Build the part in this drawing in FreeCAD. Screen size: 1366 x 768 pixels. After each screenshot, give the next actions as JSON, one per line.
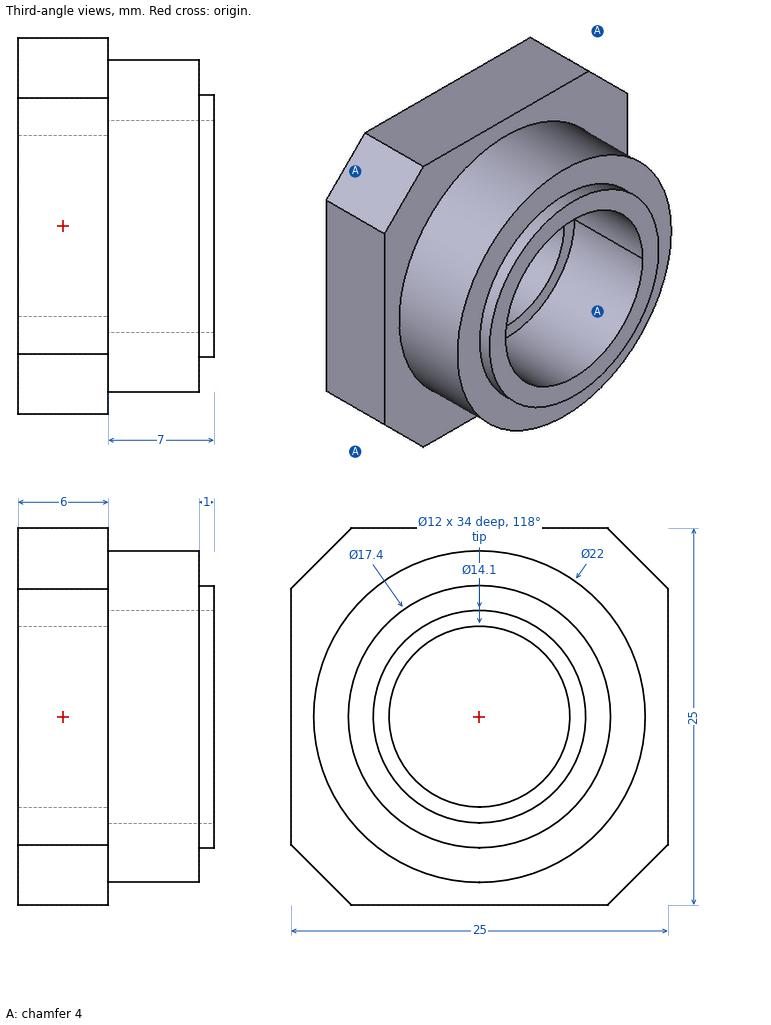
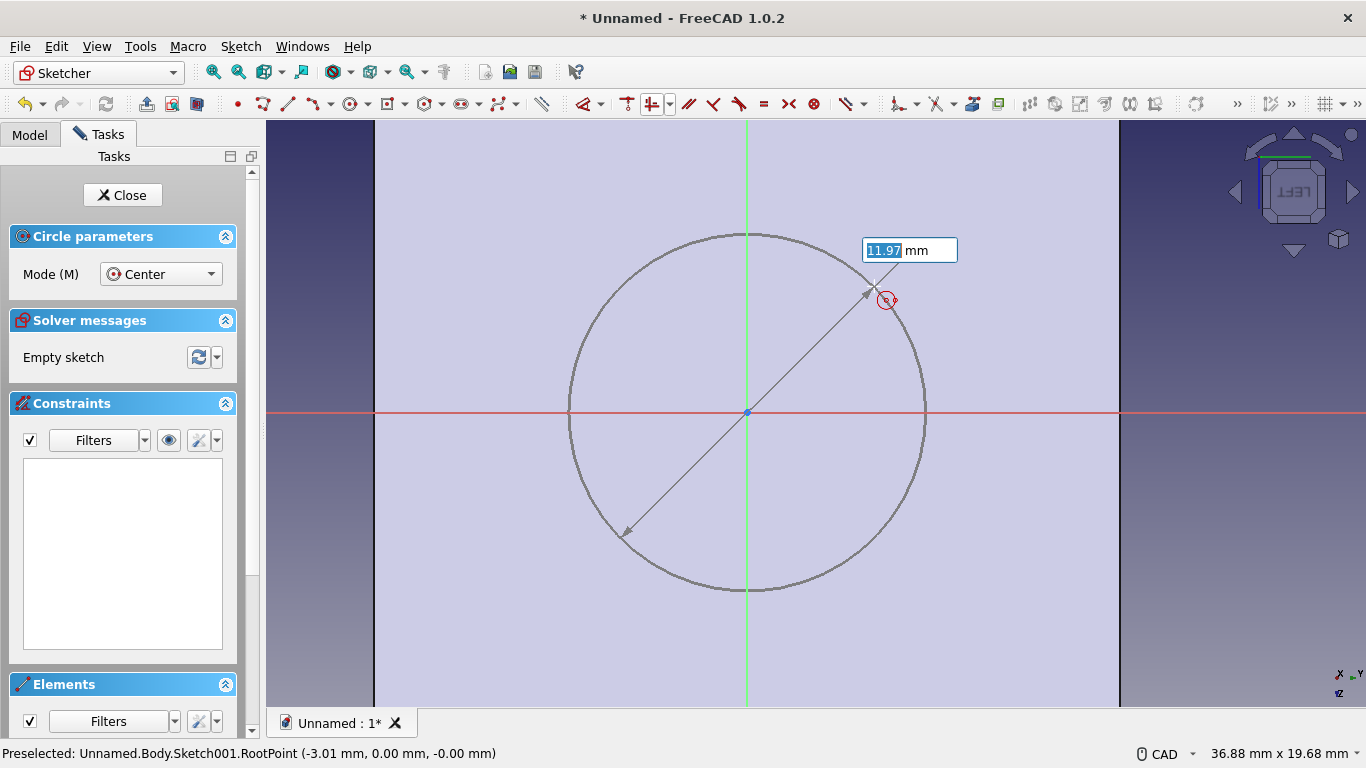
{"action": "type", "text": "12"}
{"action": "key", "text": "Return"}
{"action": "key", "text": "Escape"}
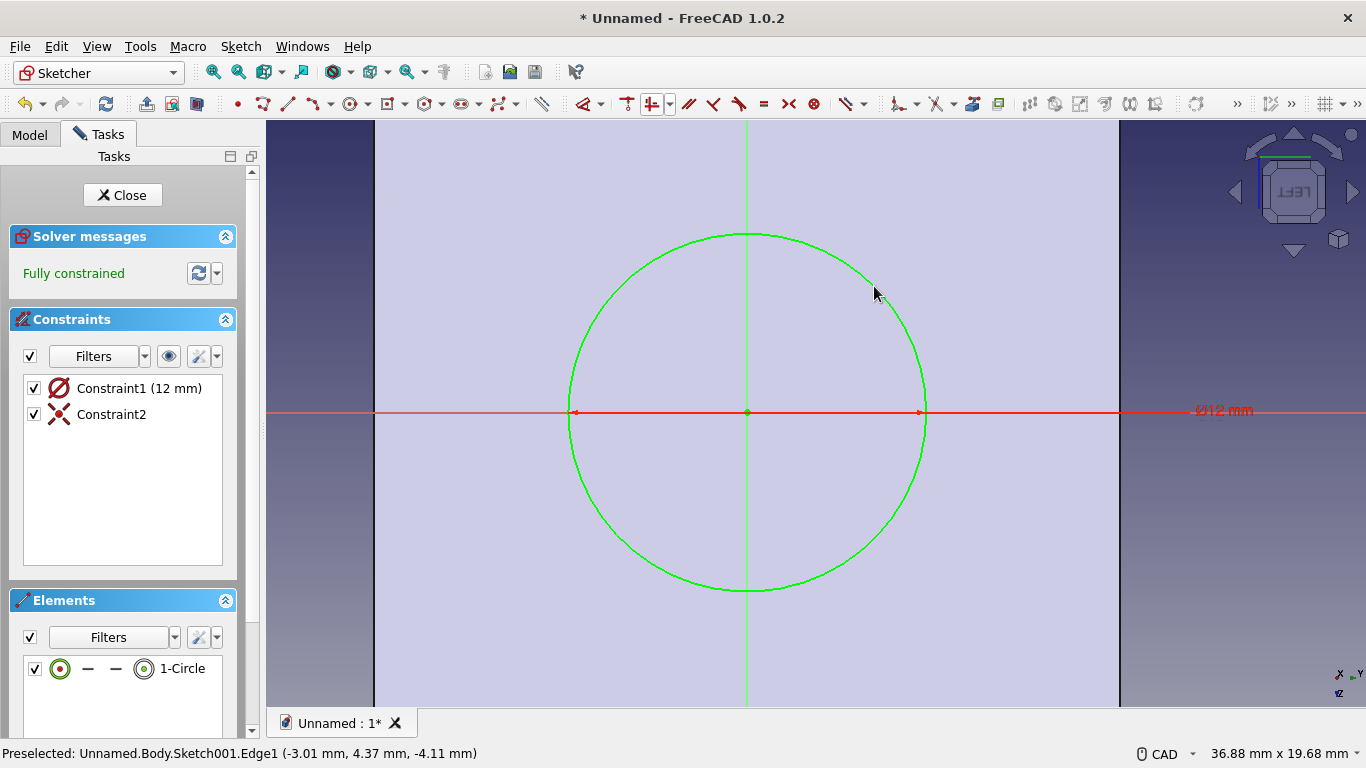
{"action": "left_click", "coordinate": [123, 195]}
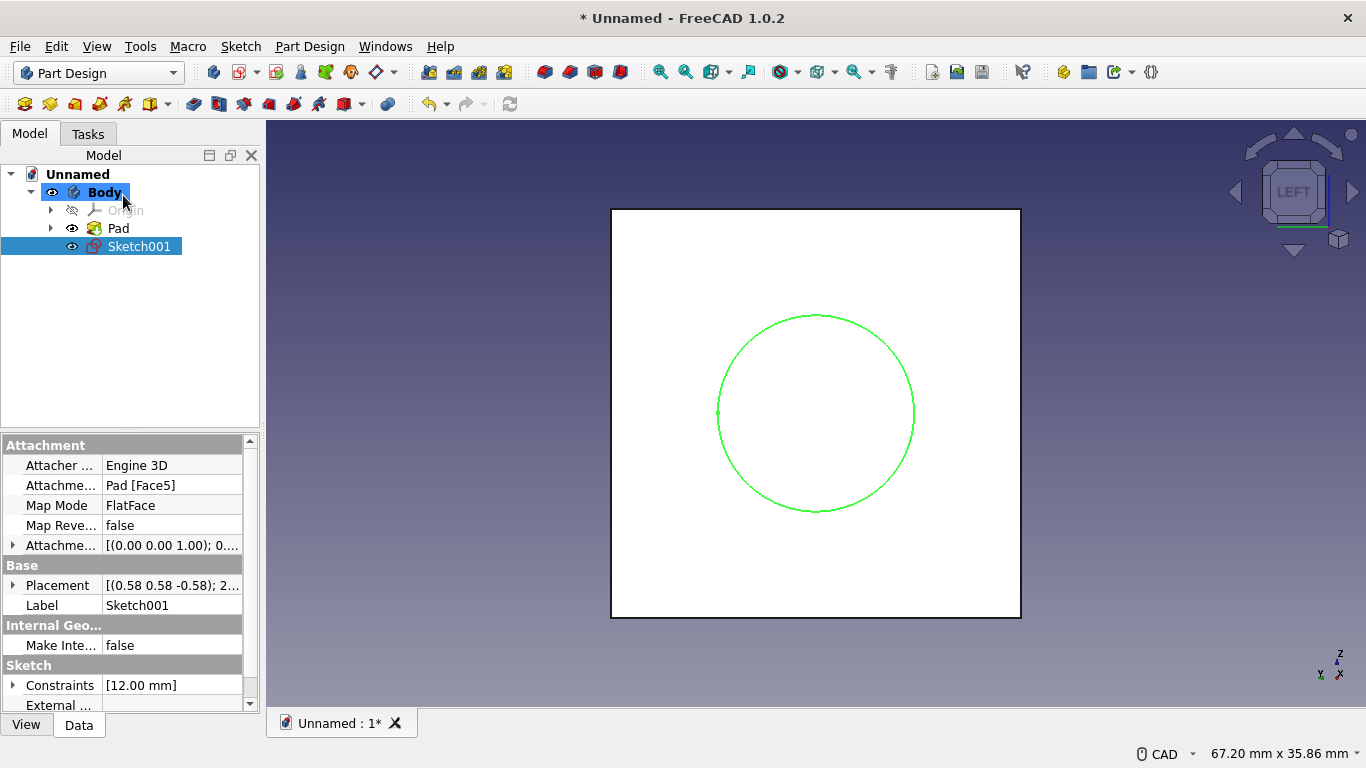
{"action": "left_click", "coordinate": [219, 104]}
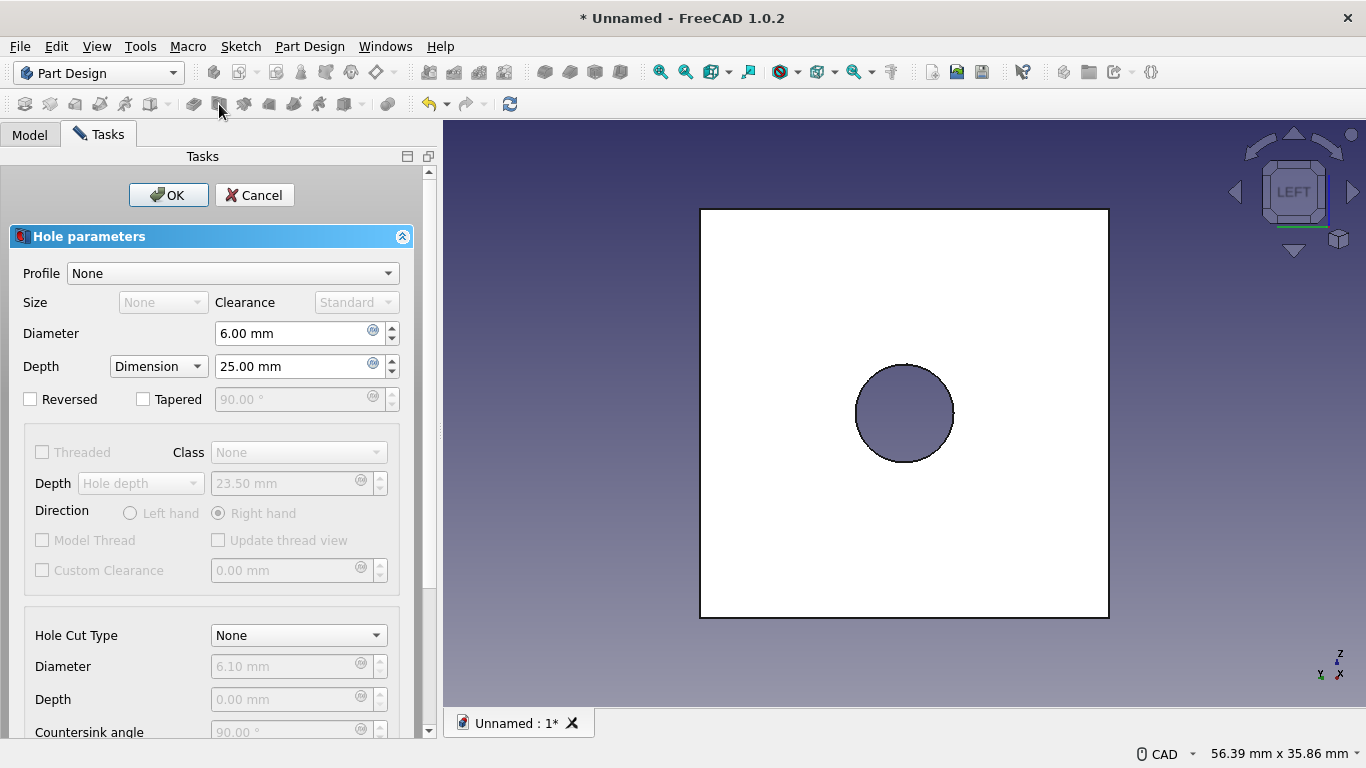
{"action": "triple_click", "coordinate": [300, 334]}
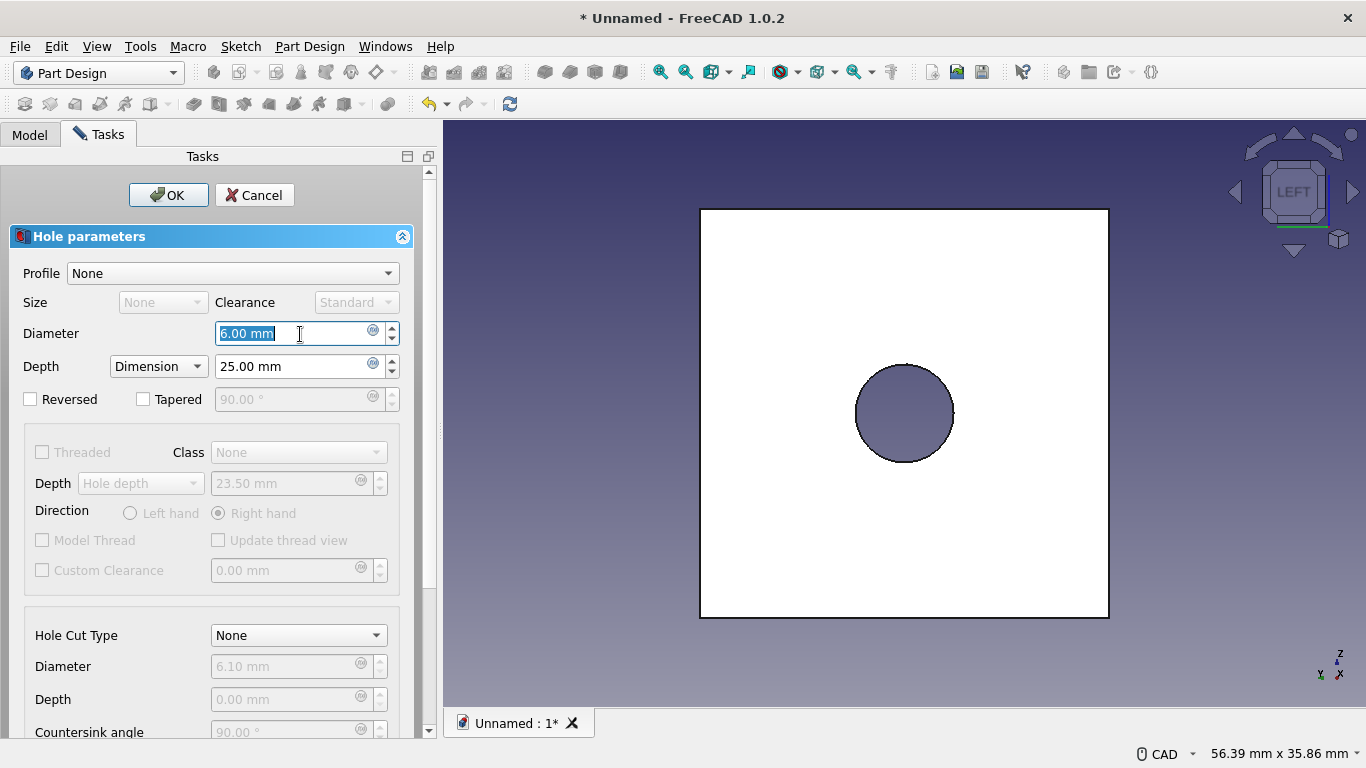
{"action": "type", "text": "12"}
{"action": "key", "text": "Tab"}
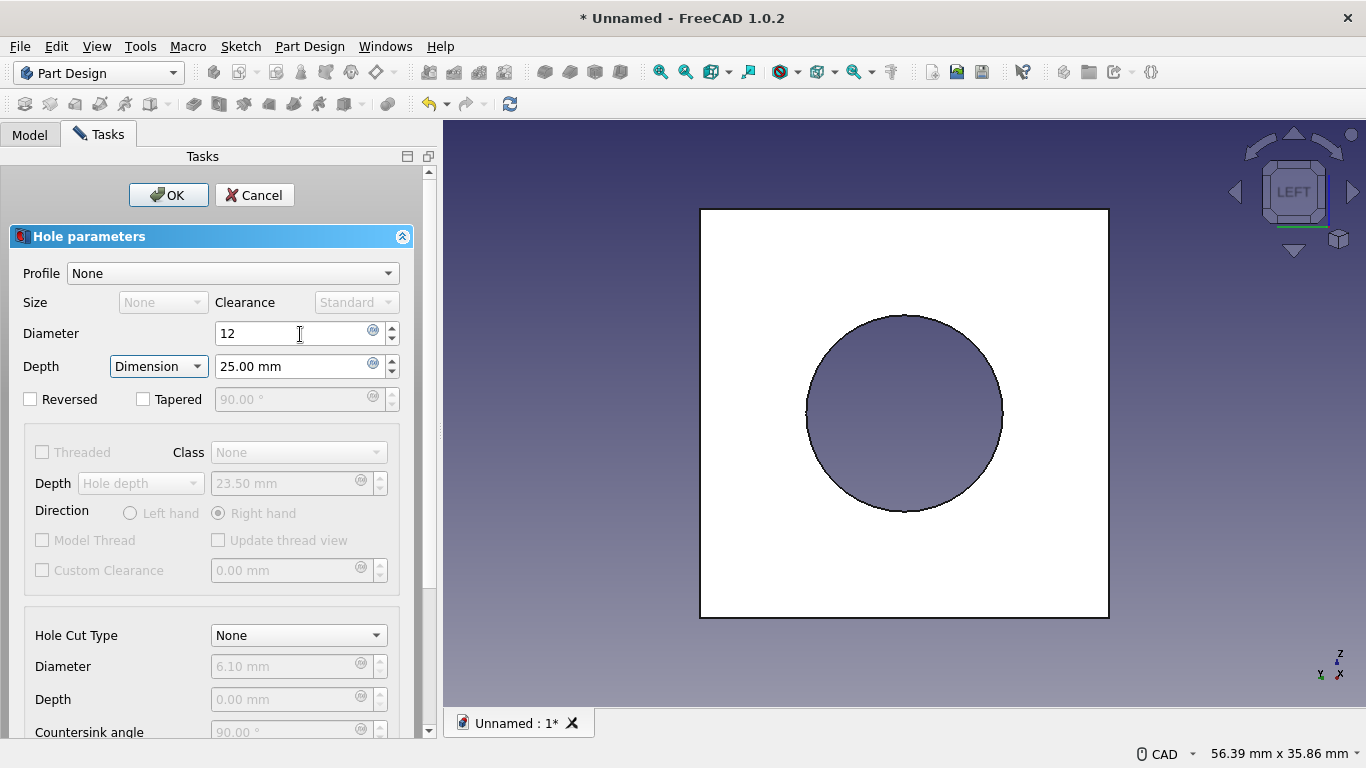
{"action": "triple_click", "coordinate": [300, 366]}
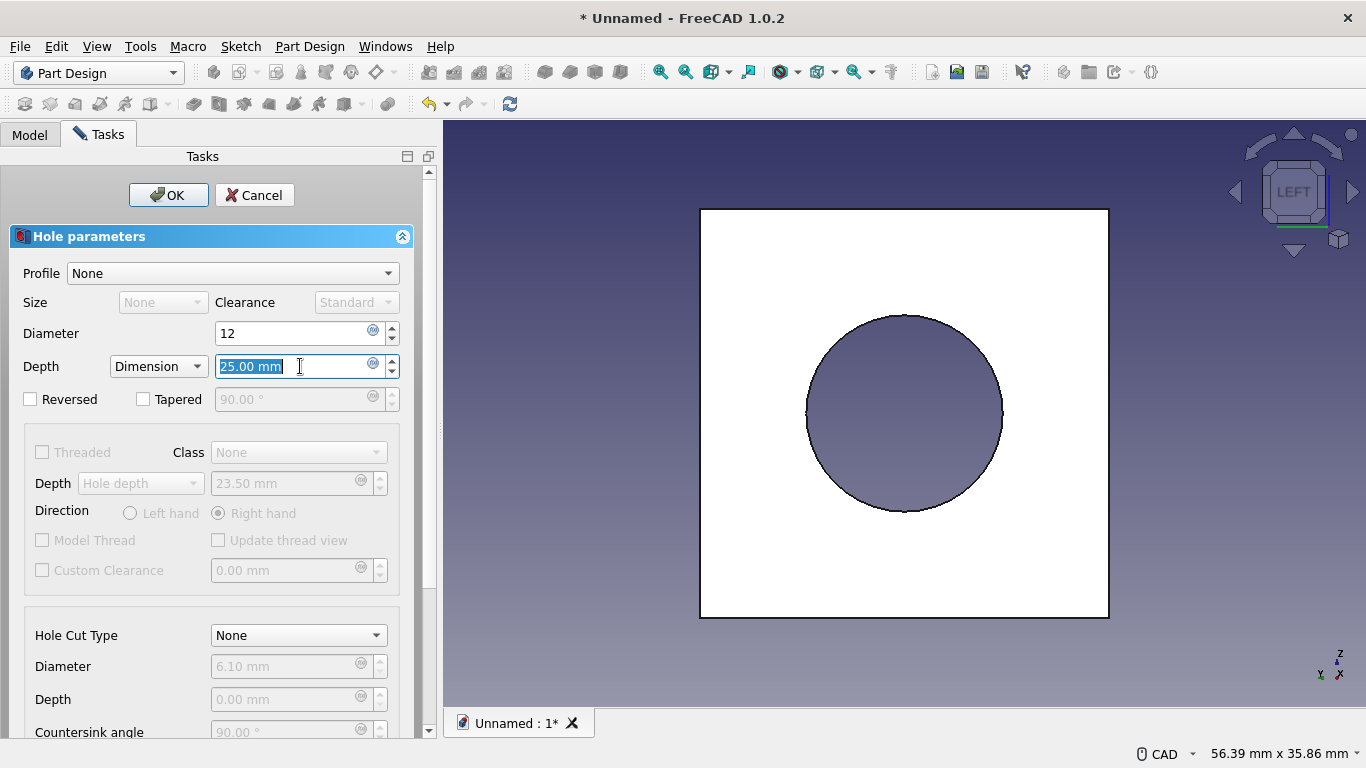
{"action": "type", "text": "34"}
{"action": "key", "text": "Tab"}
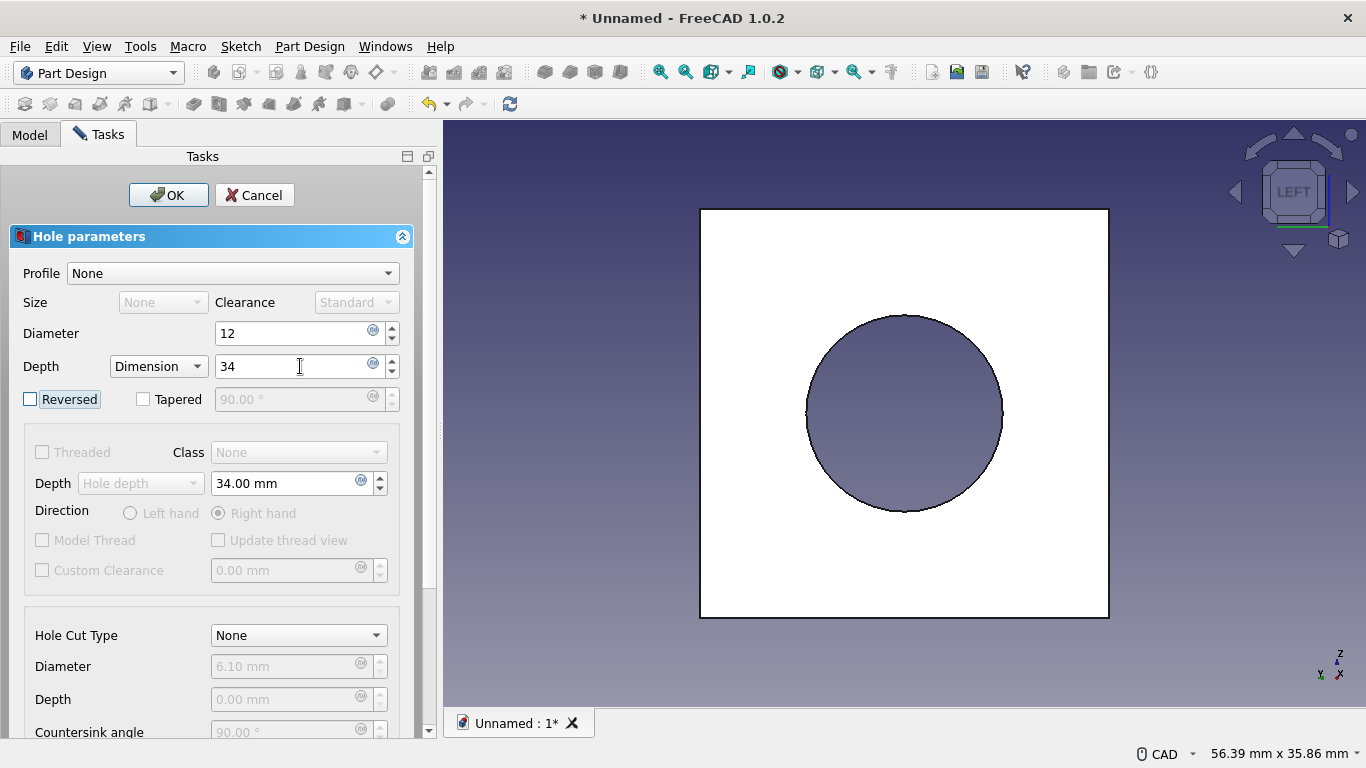
{"action": "left_click", "coordinate": [169, 195]}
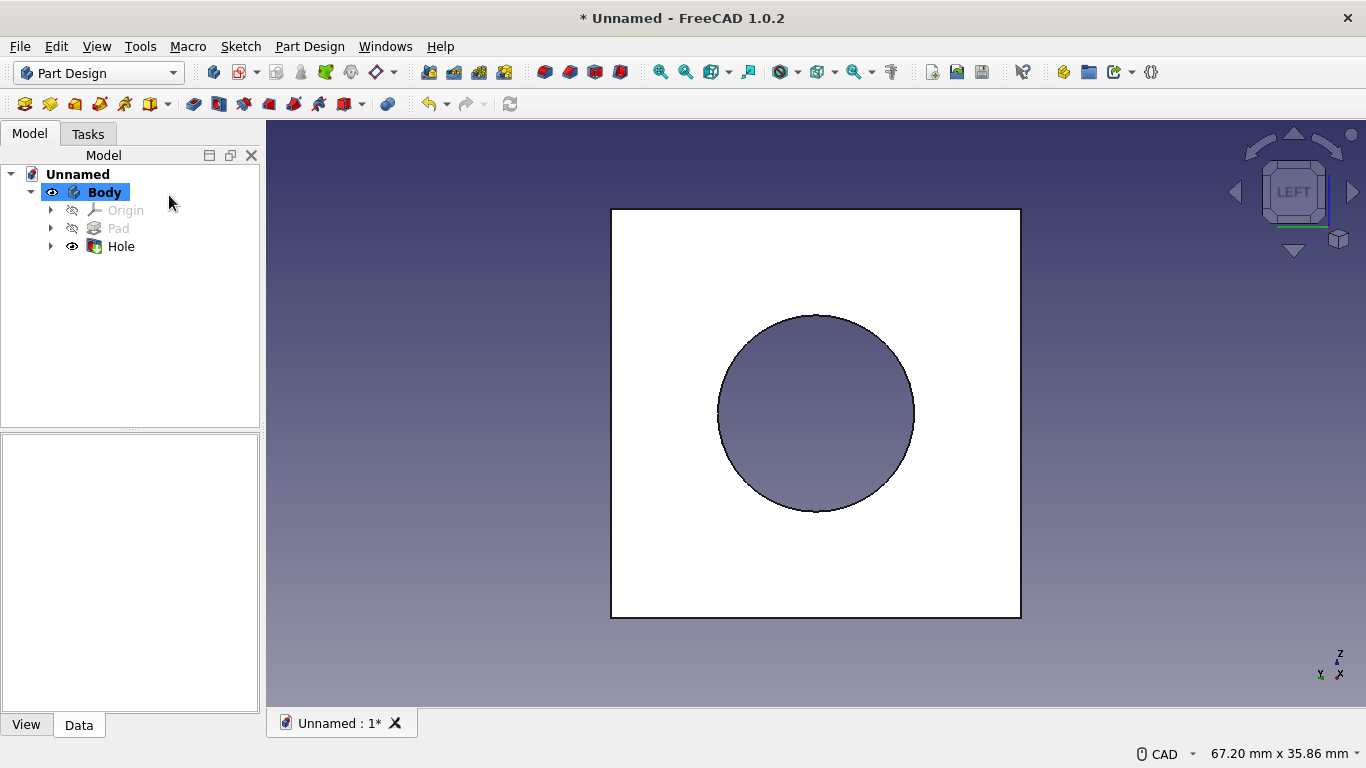
{"action": "key", "text": "0"}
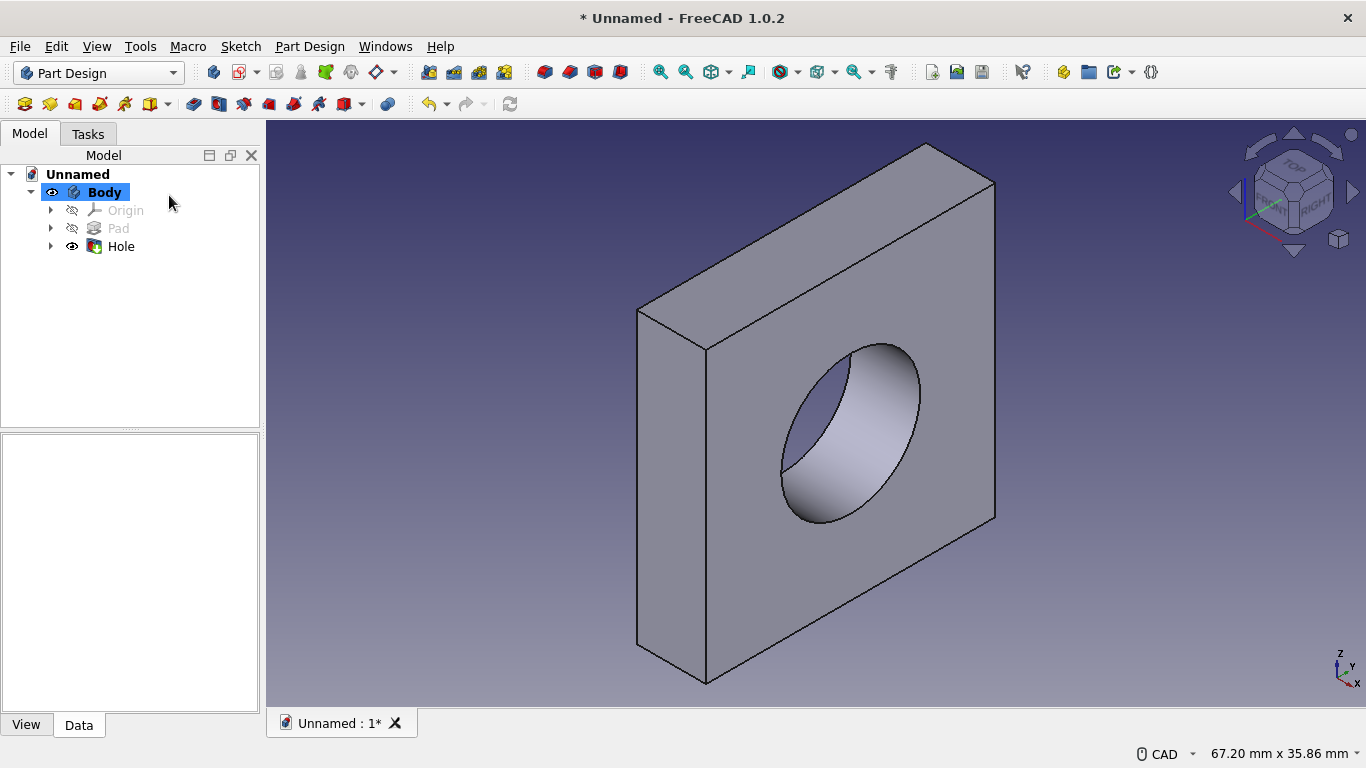
{"action": "left_click", "coordinate": [768, 385]}